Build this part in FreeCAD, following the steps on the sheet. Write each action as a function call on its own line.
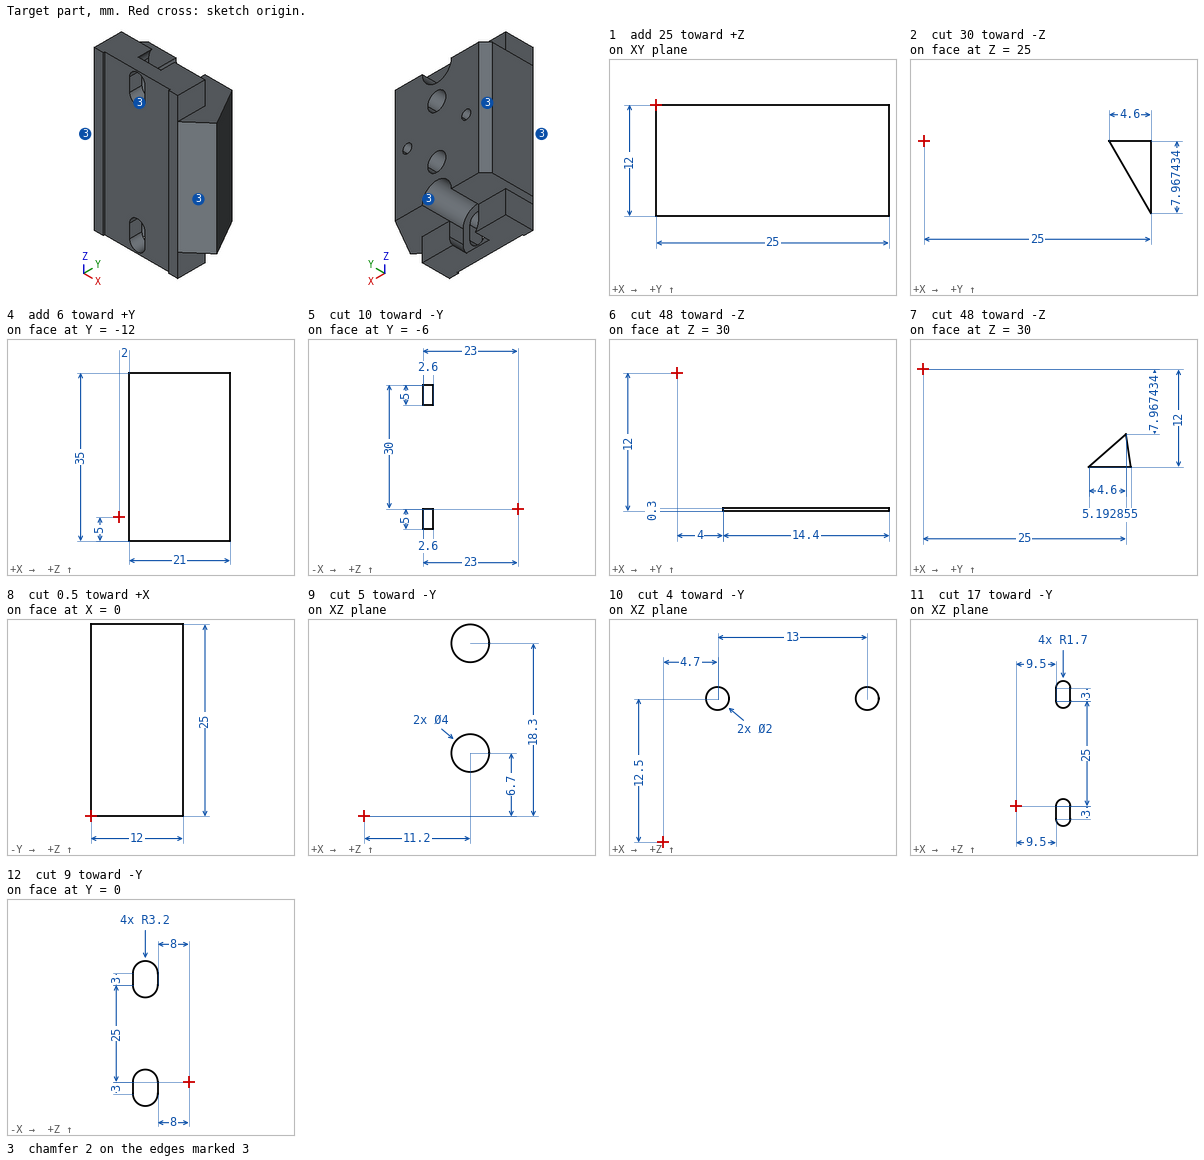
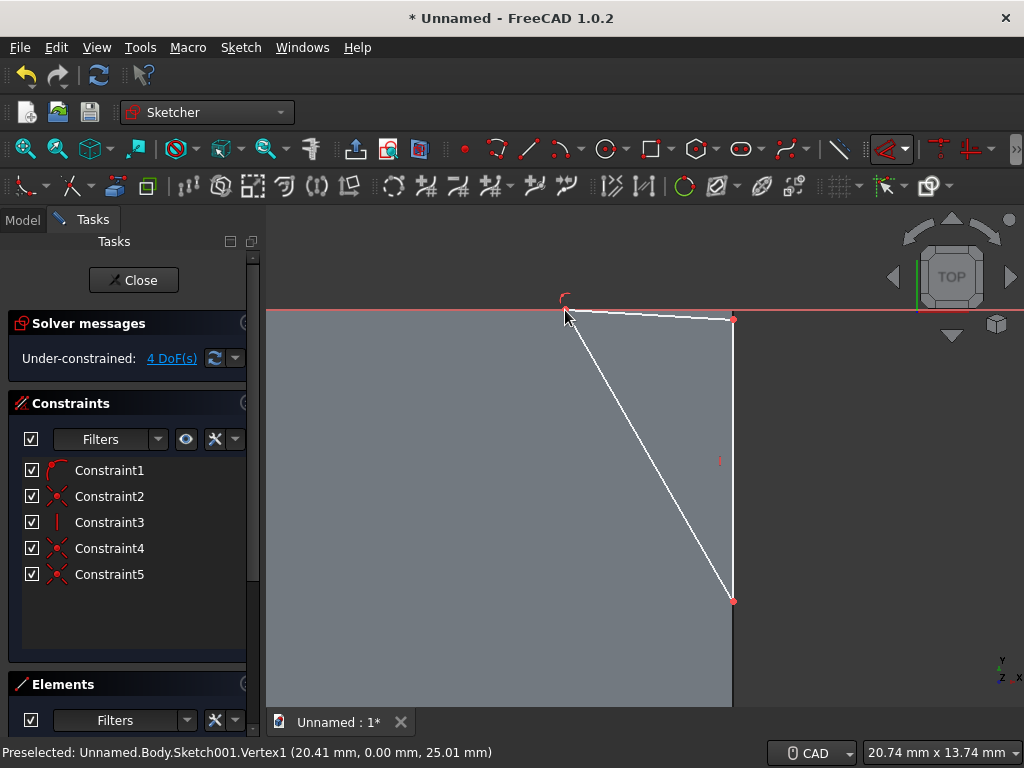
click(615, 313)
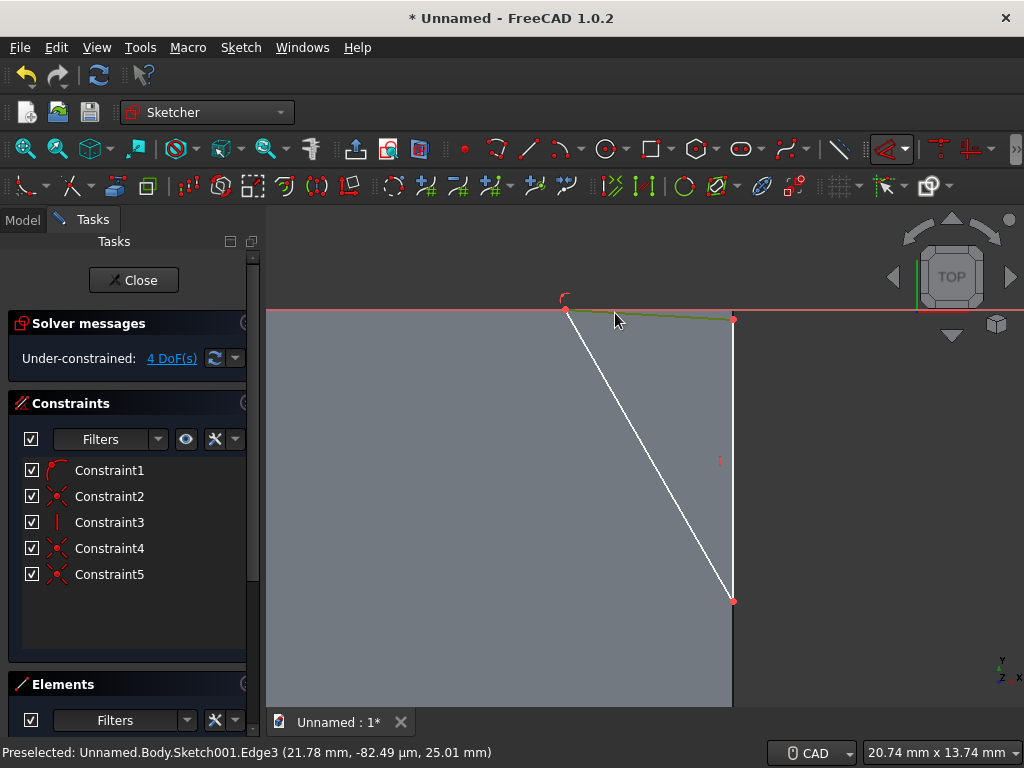
key(h)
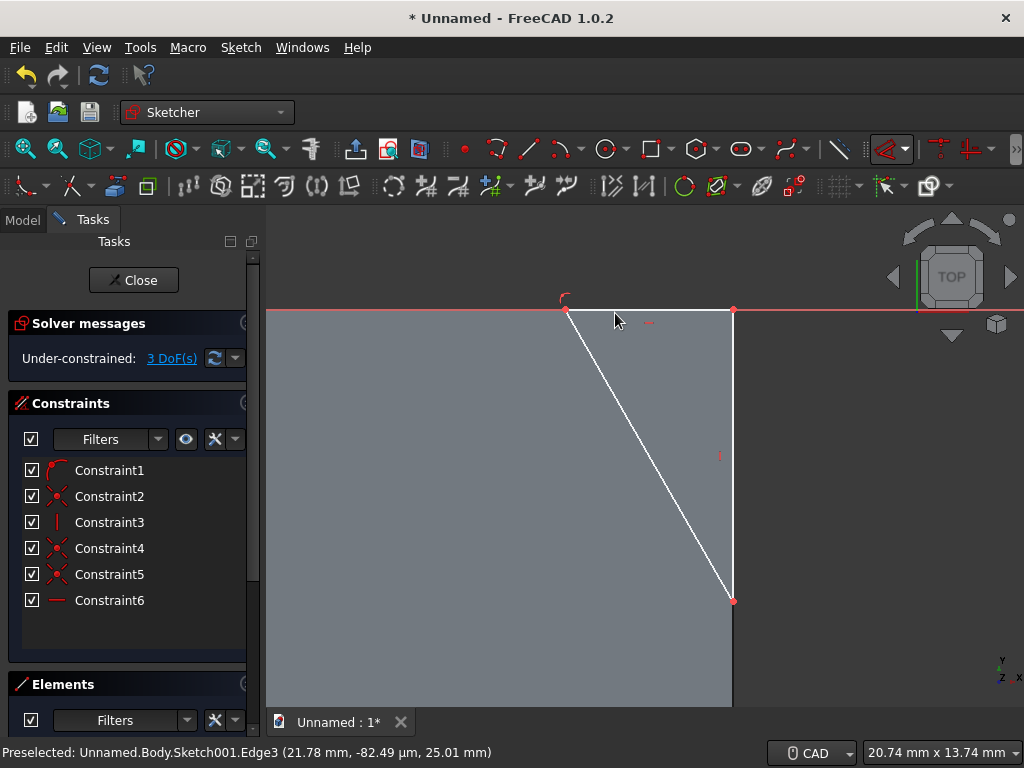
click(683, 310)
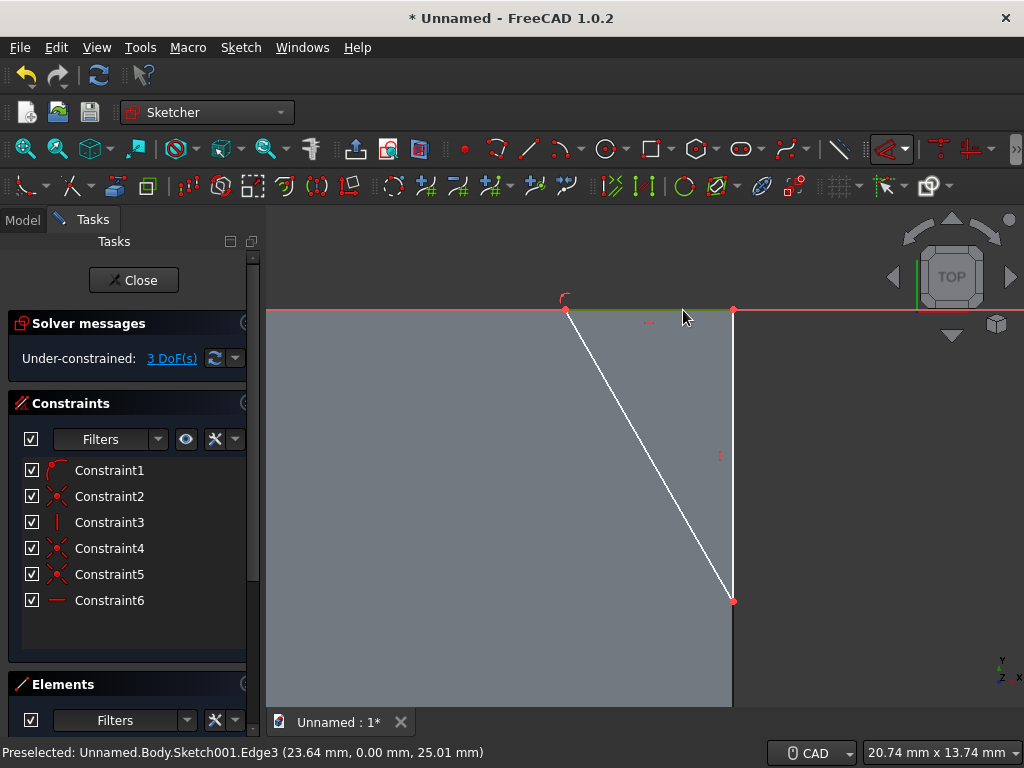
key(l)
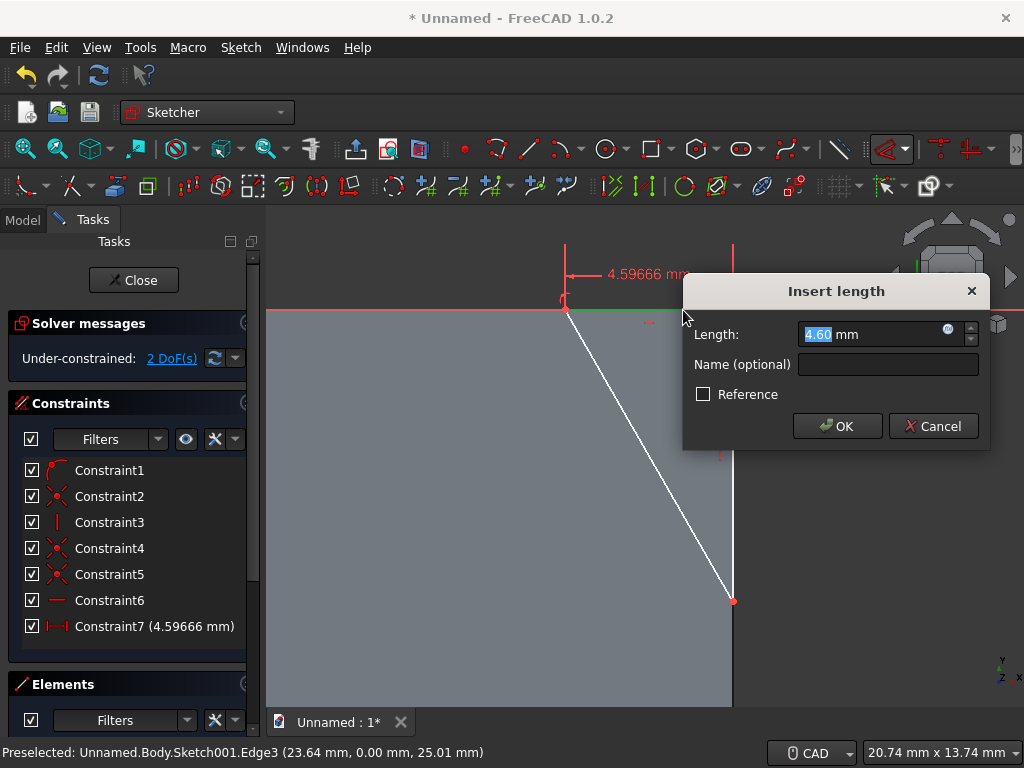
text(4.6)
key(Return)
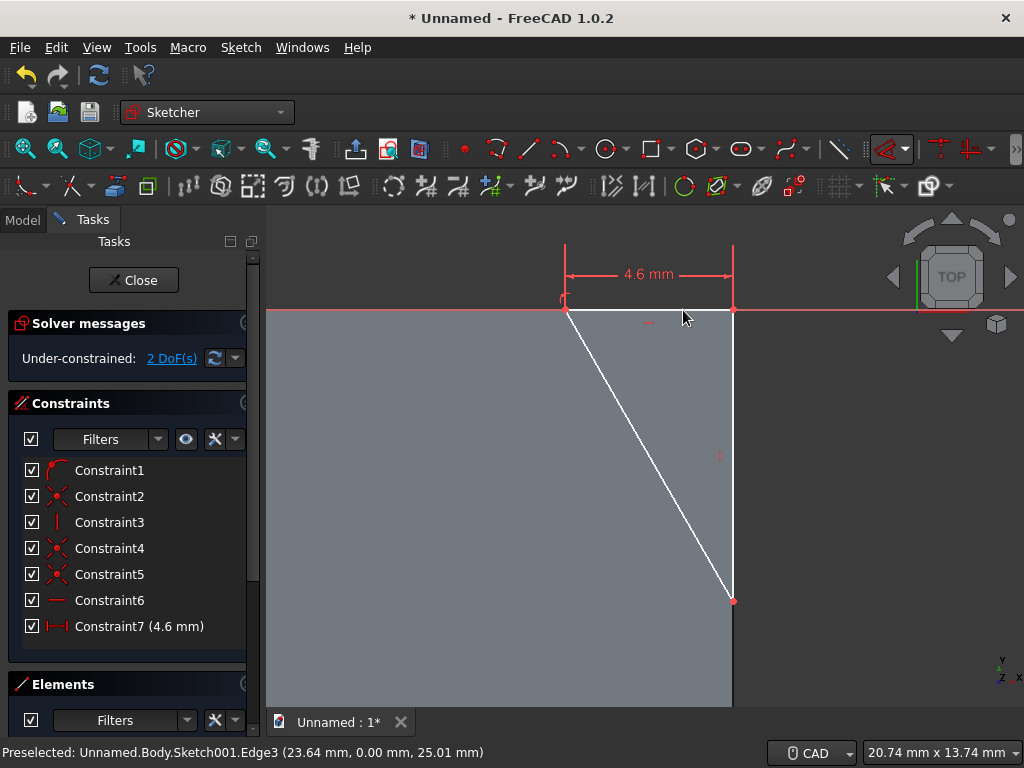
click(733, 602)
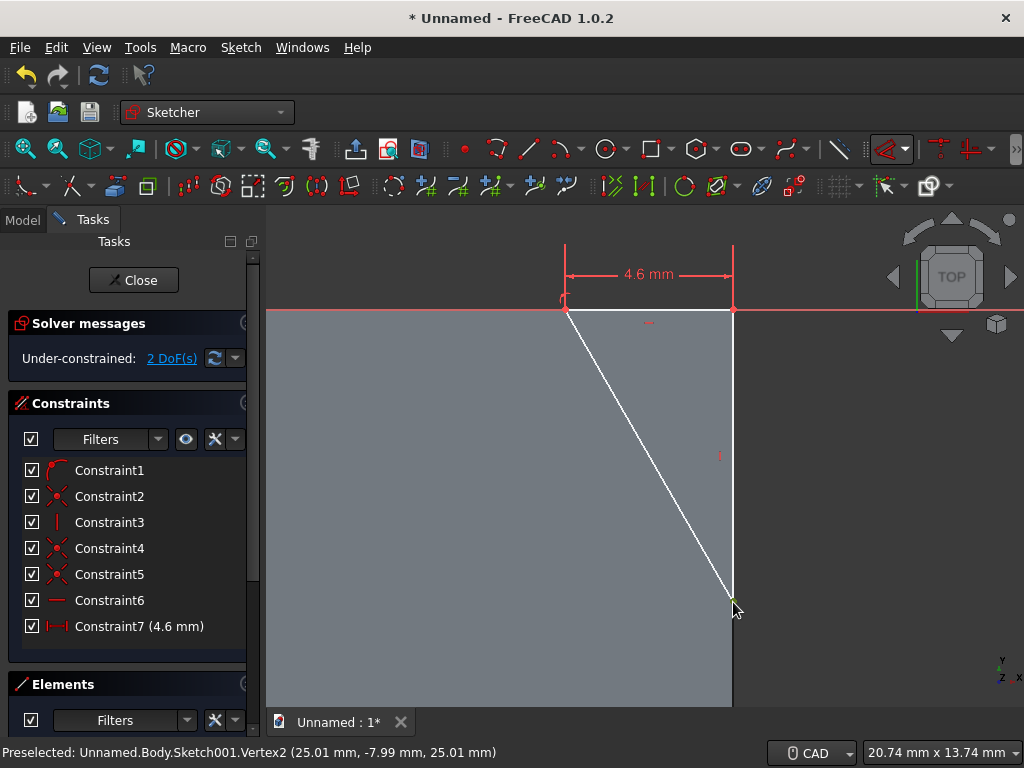
click(908, 150)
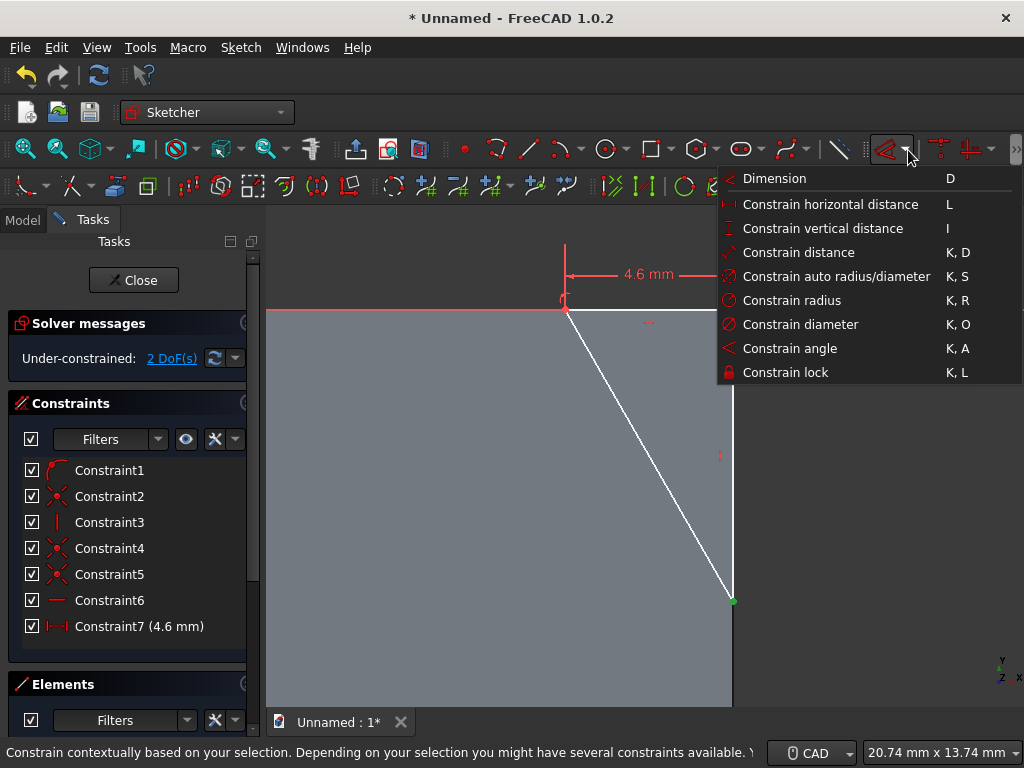
click(870, 204)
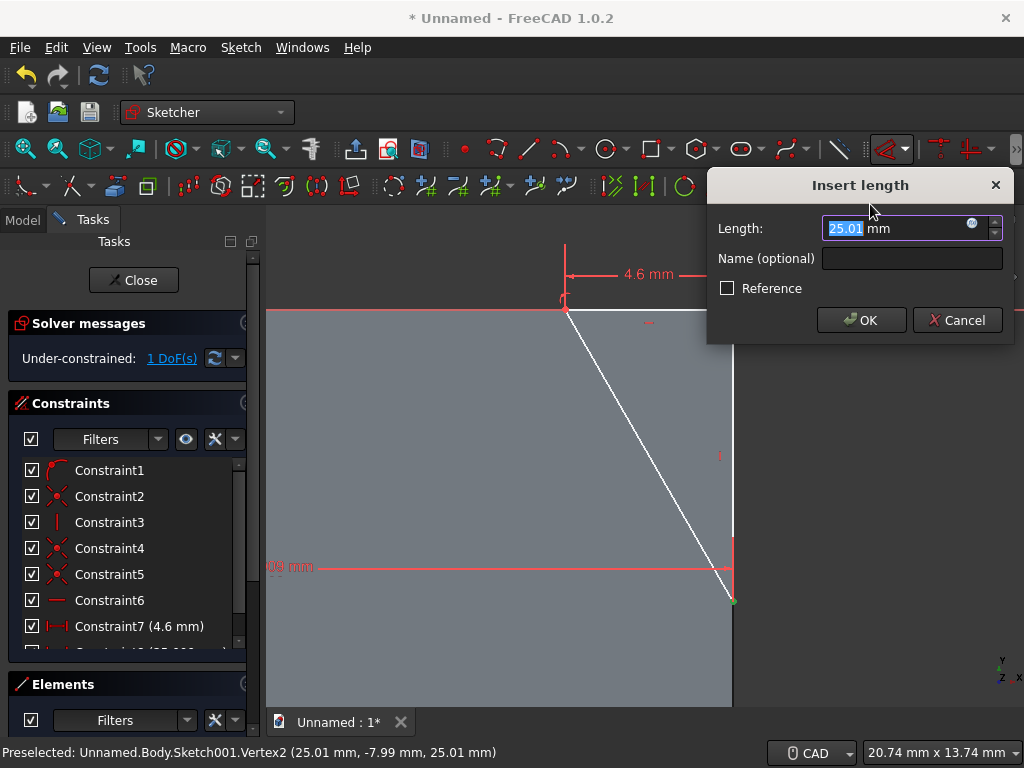
text(25)
key(Return)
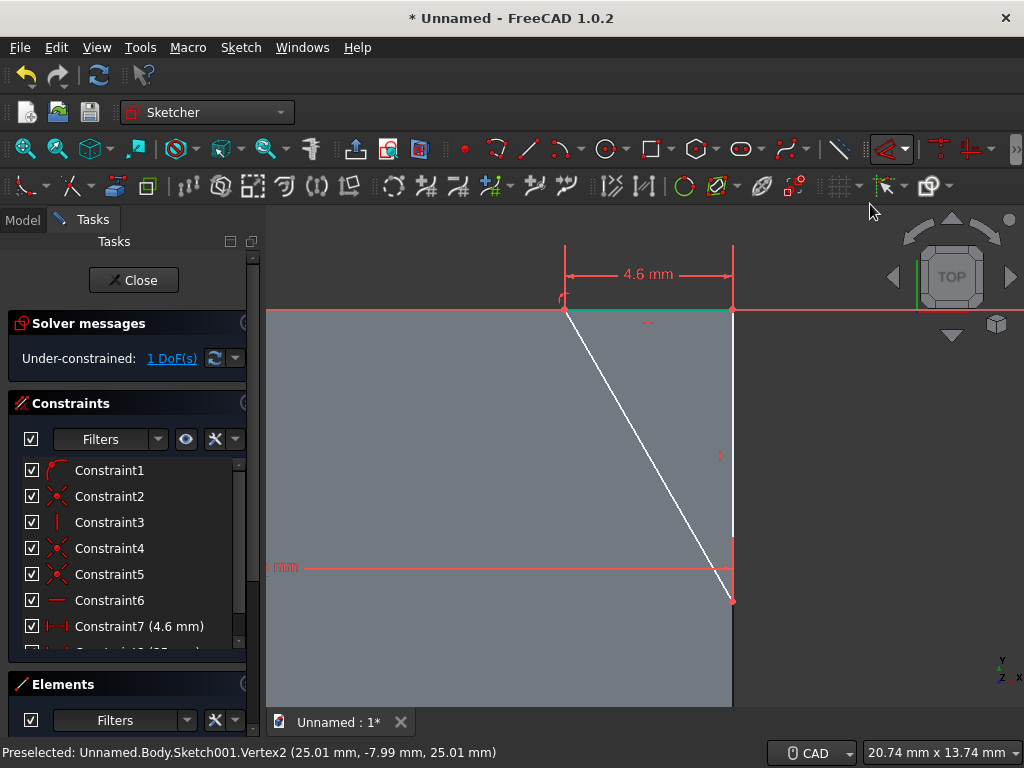
click(733, 514)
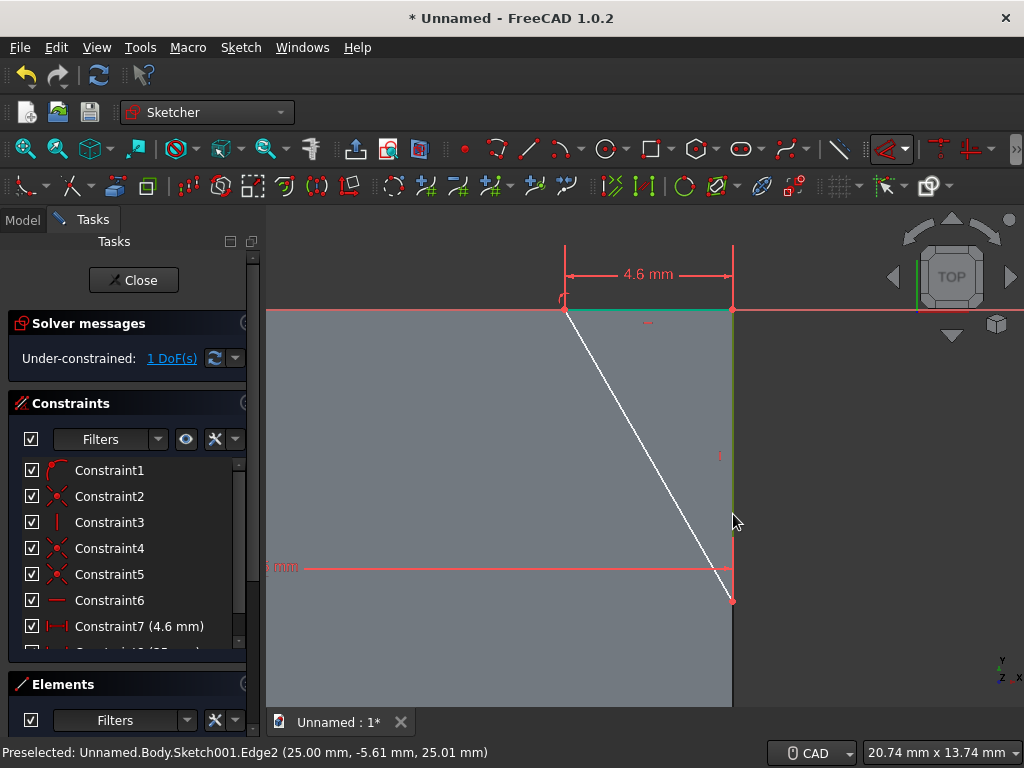
click(908, 150)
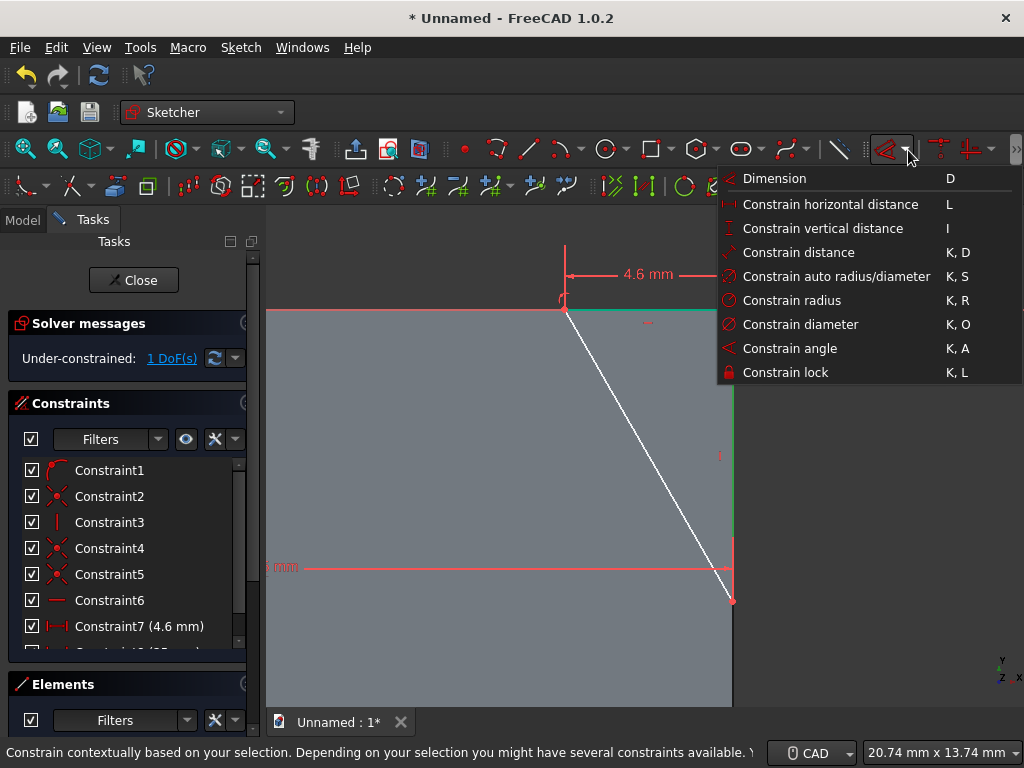
click(870, 228)